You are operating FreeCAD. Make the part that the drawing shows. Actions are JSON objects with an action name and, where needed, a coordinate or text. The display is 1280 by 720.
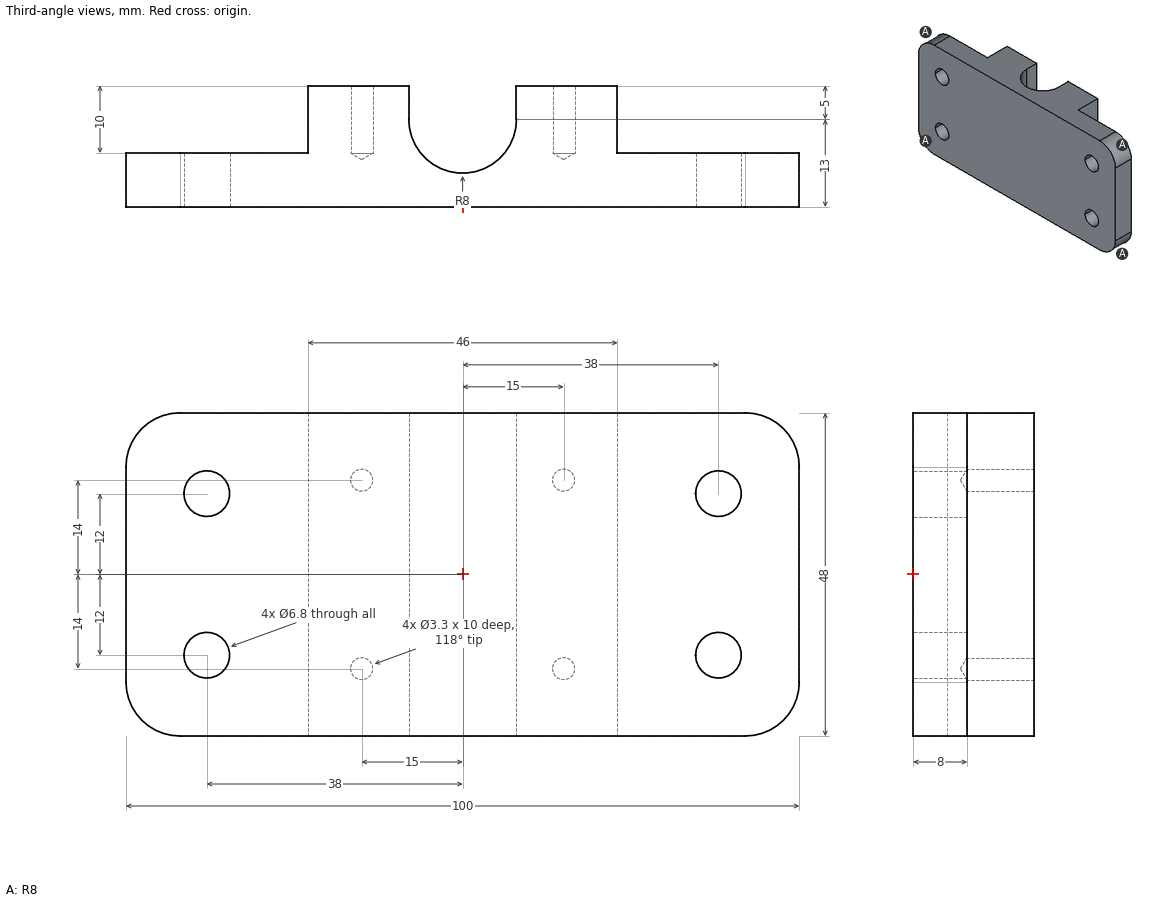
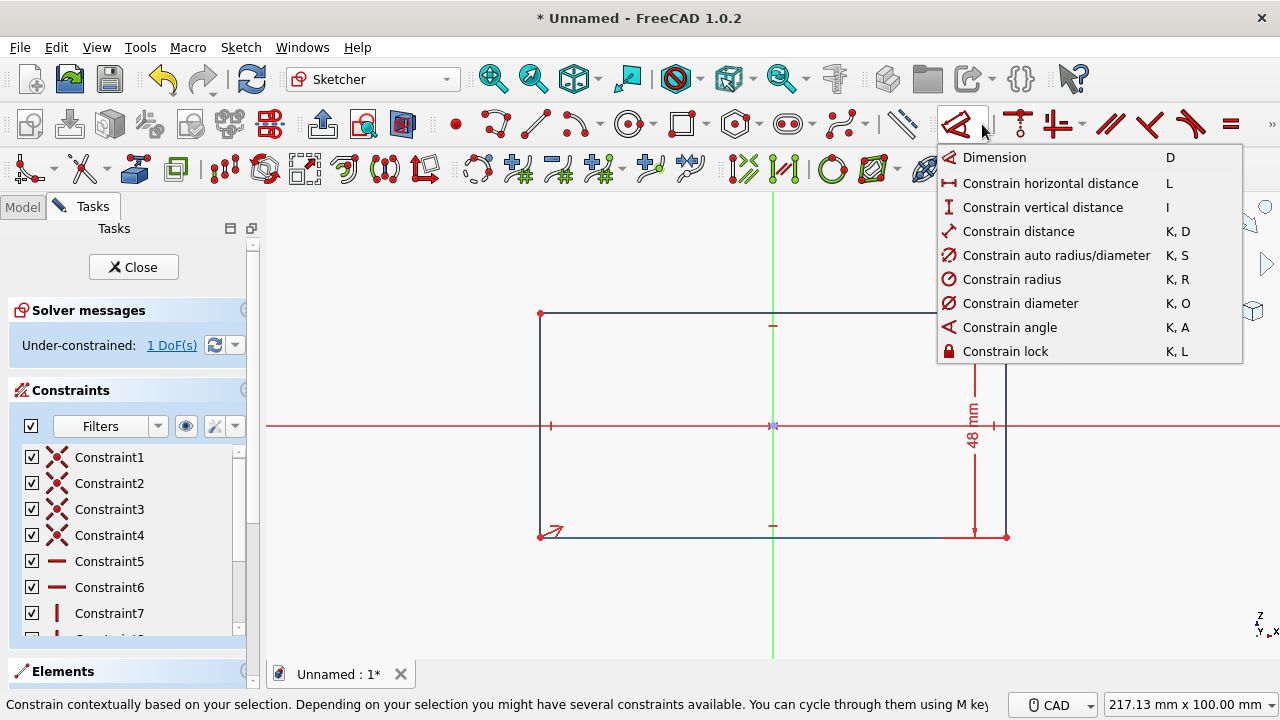
{"action": "left_click", "coordinate": [1090, 183]}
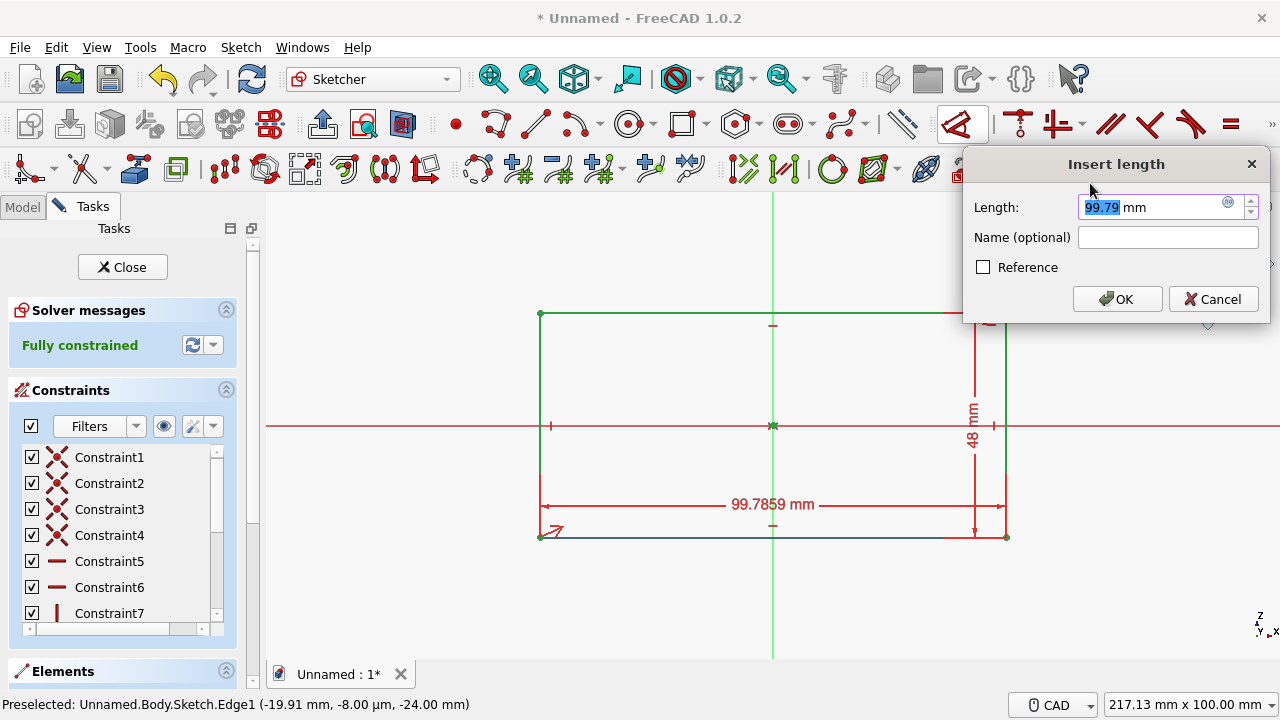
{"action": "type", "text": "100"}
{"action": "key", "text": "Return"}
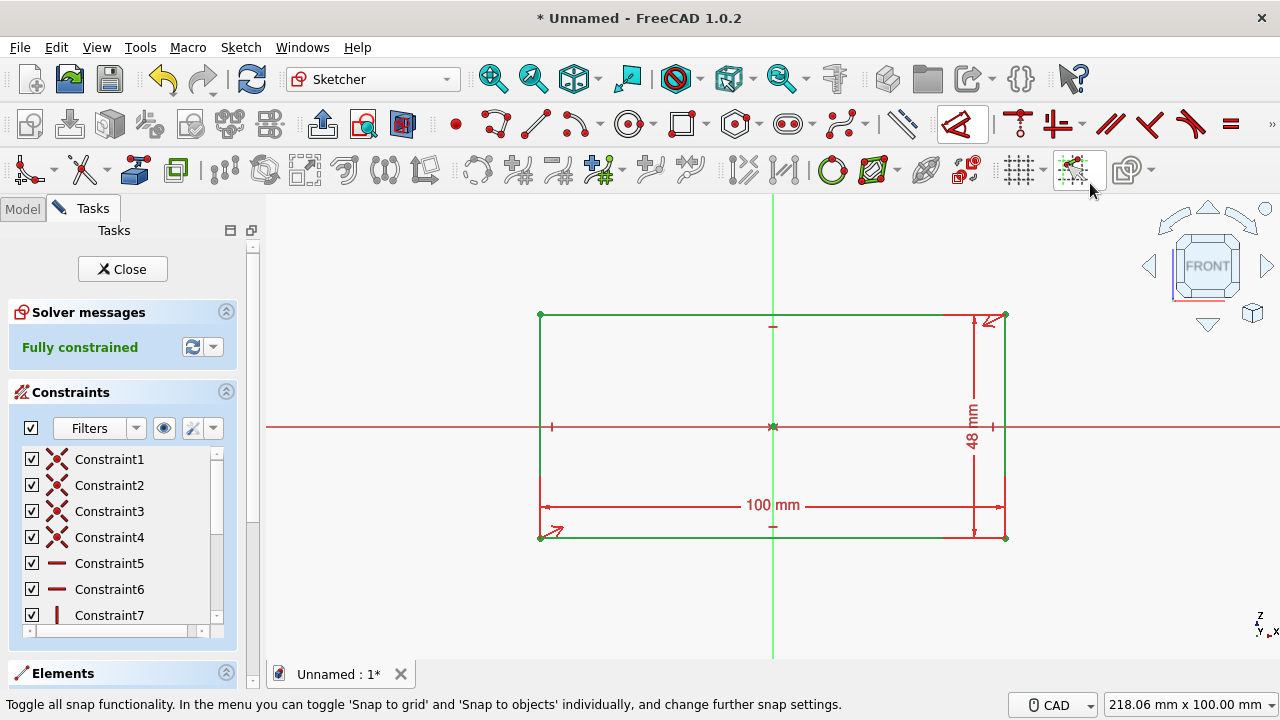
{"action": "left_click", "coordinate": [123, 269]}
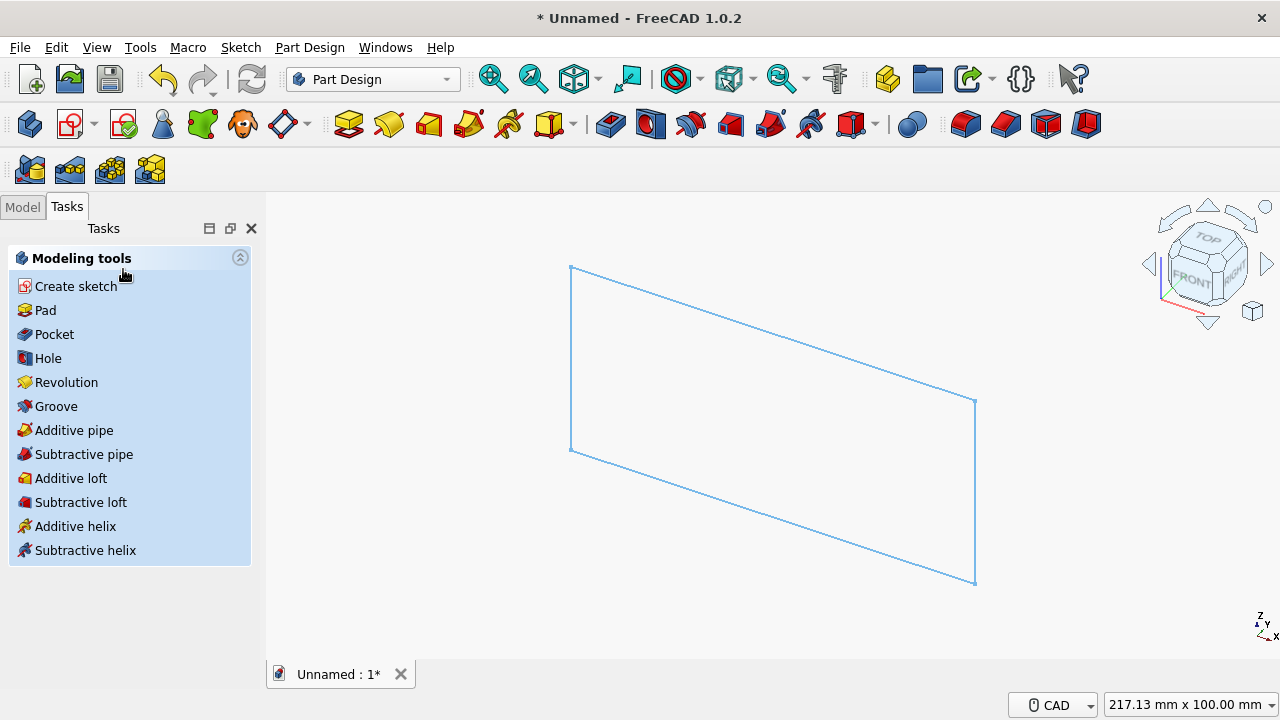
{"action": "left_click", "coordinate": [350, 124]}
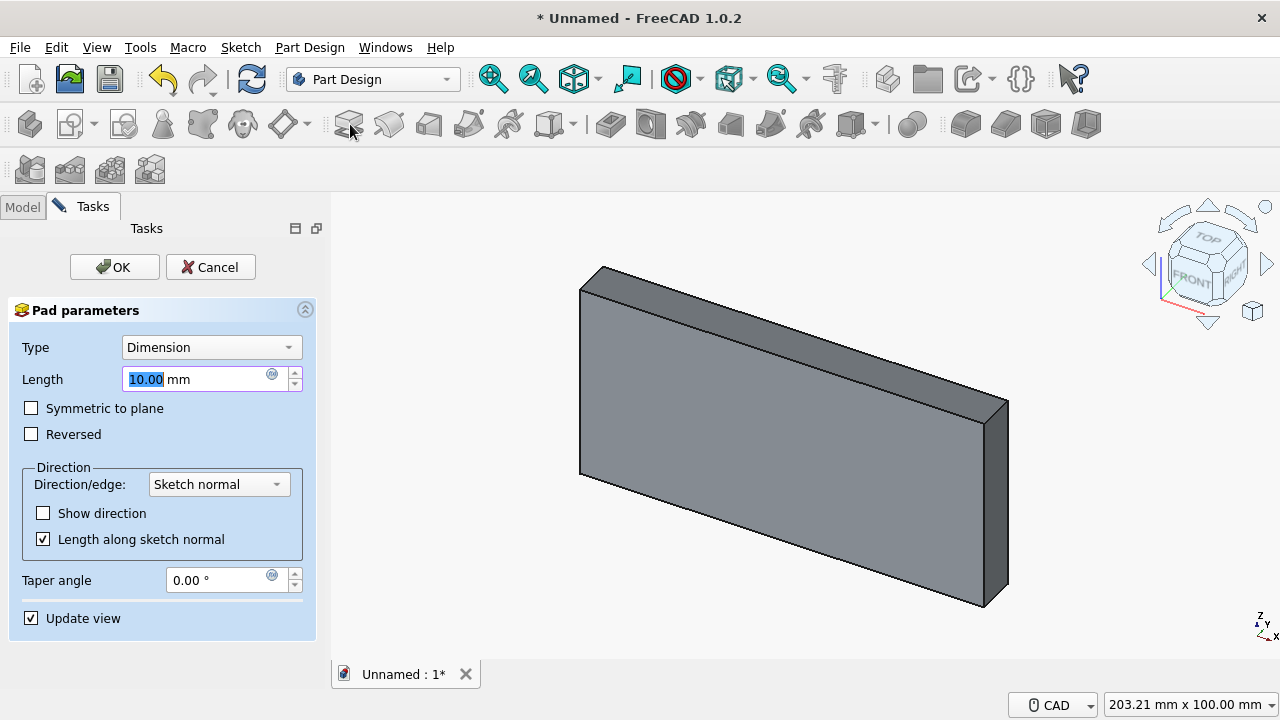
{"action": "type", "text": "8"}
{"action": "key", "text": "Tab"}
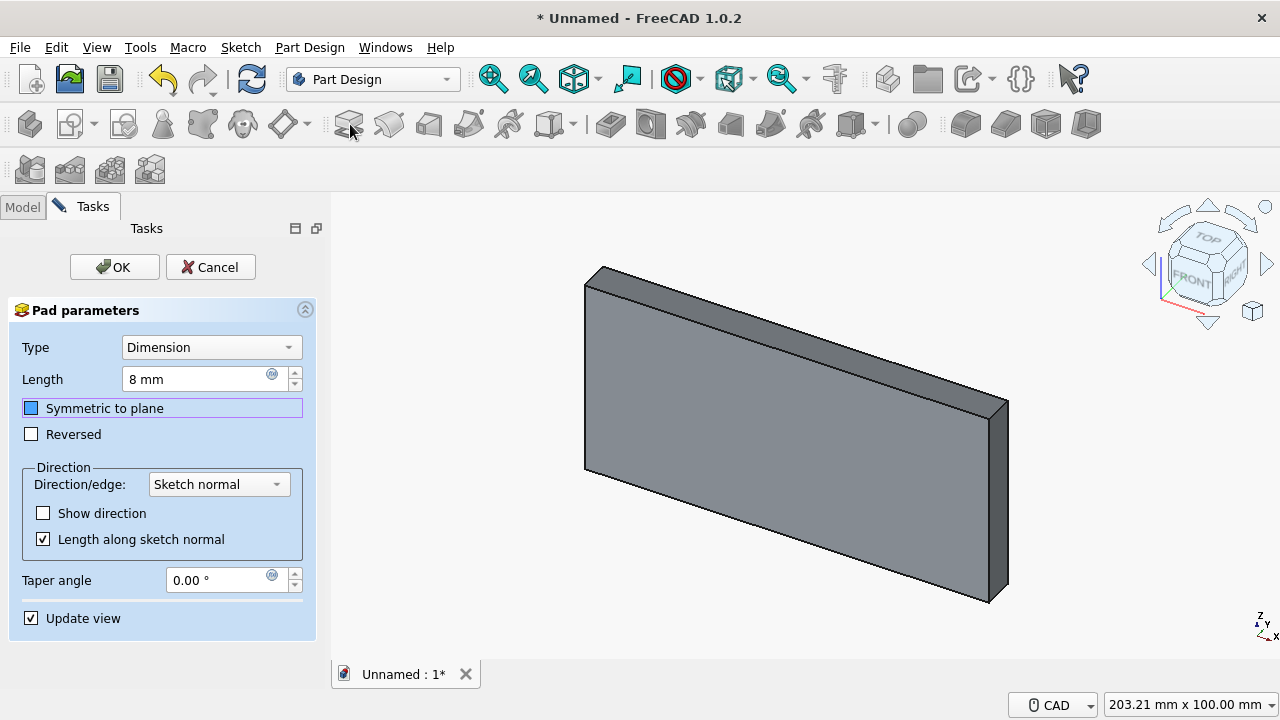
{"action": "left_click", "coordinate": [30, 434]}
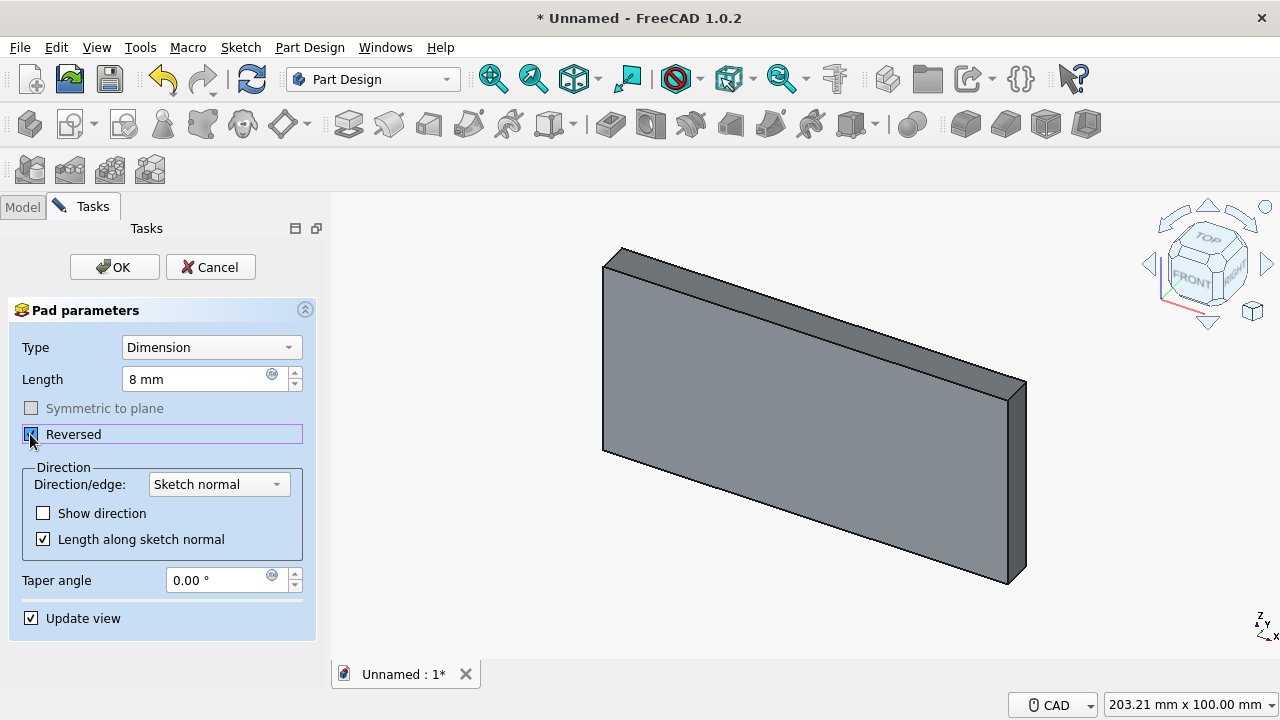
{"action": "left_click", "coordinate": [115, 267]}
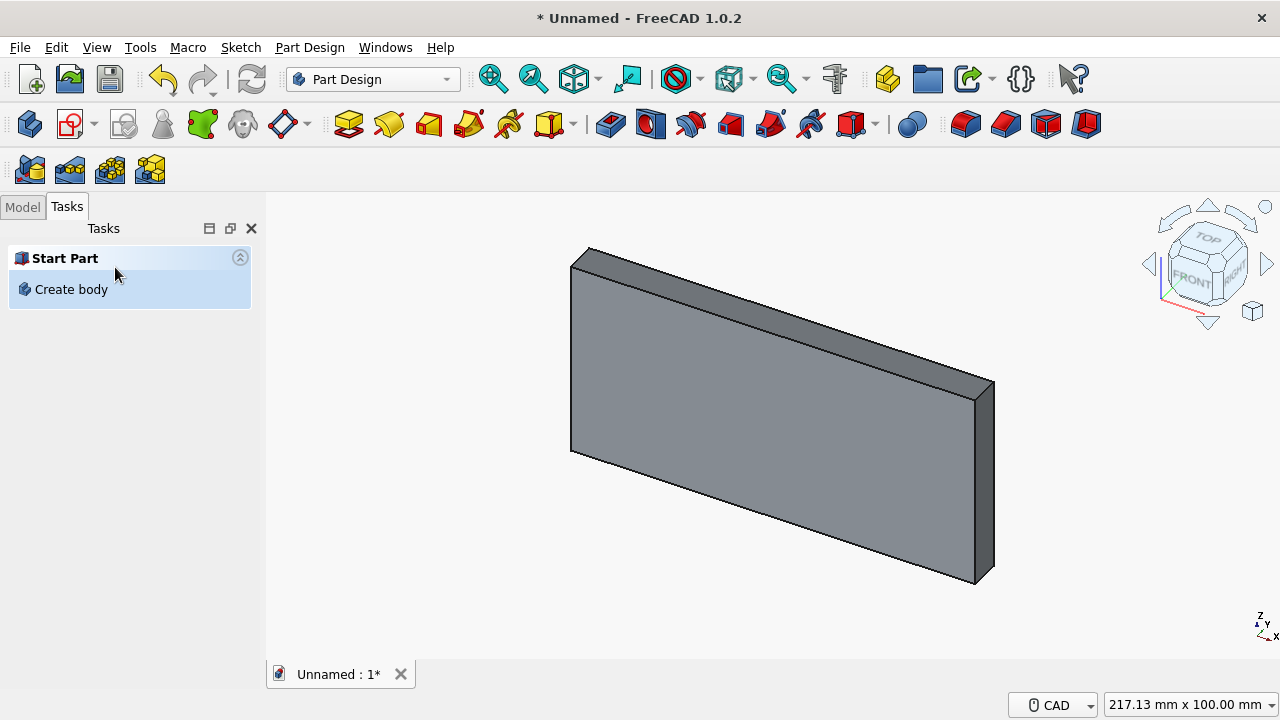
{"action": "key", "text": "4"}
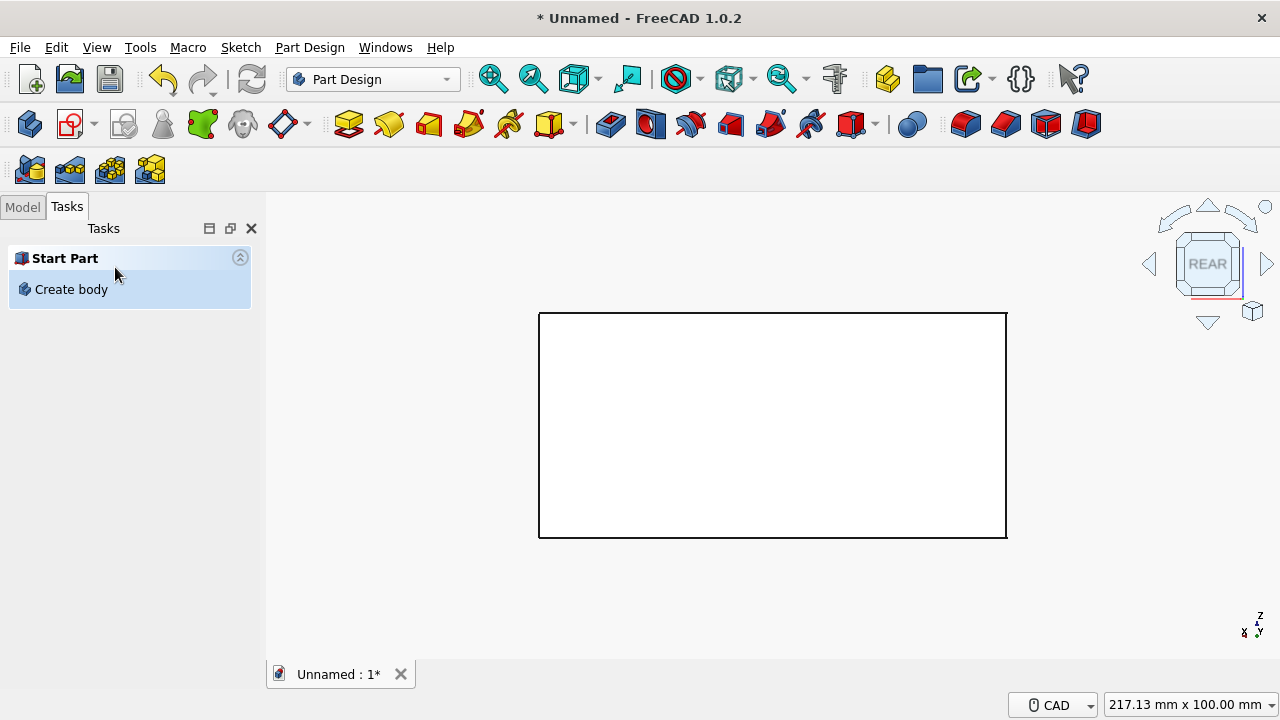
{"action": "left_click", "coordinate": [706, 424]}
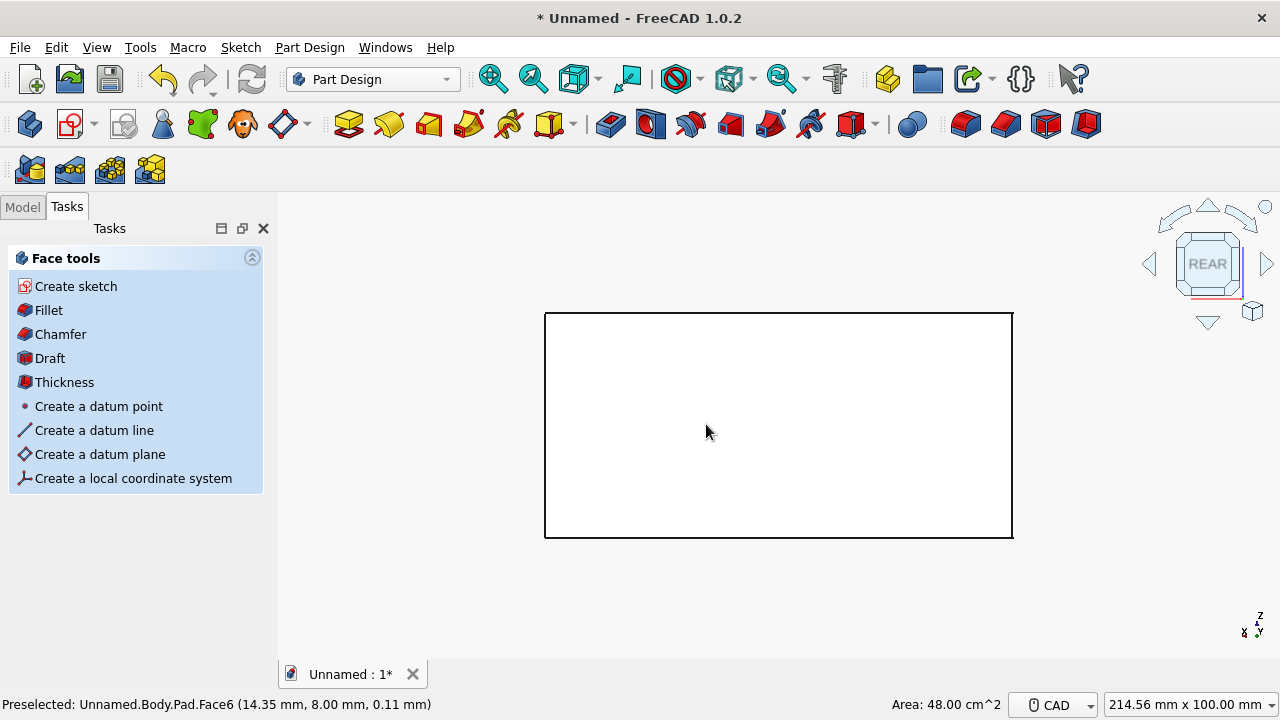
{"action": "left_click", "coordinate": [70, 124]}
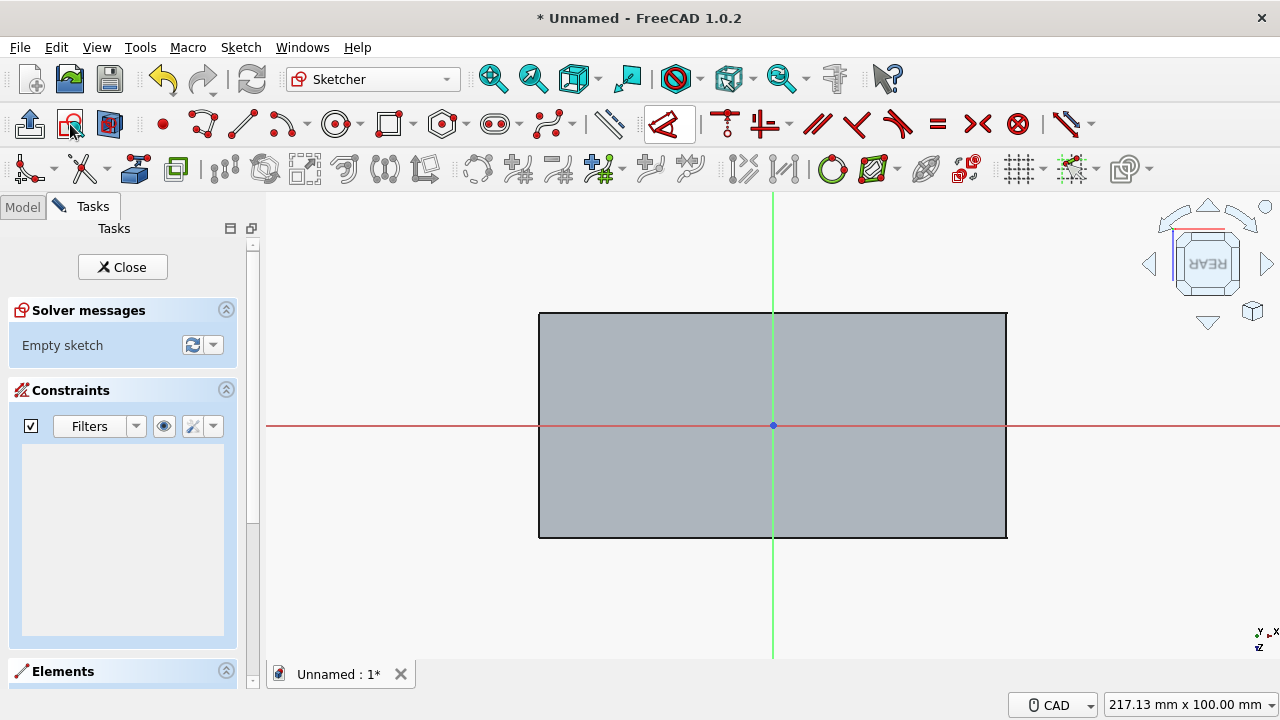
{"action": "key", "text": "g v"}